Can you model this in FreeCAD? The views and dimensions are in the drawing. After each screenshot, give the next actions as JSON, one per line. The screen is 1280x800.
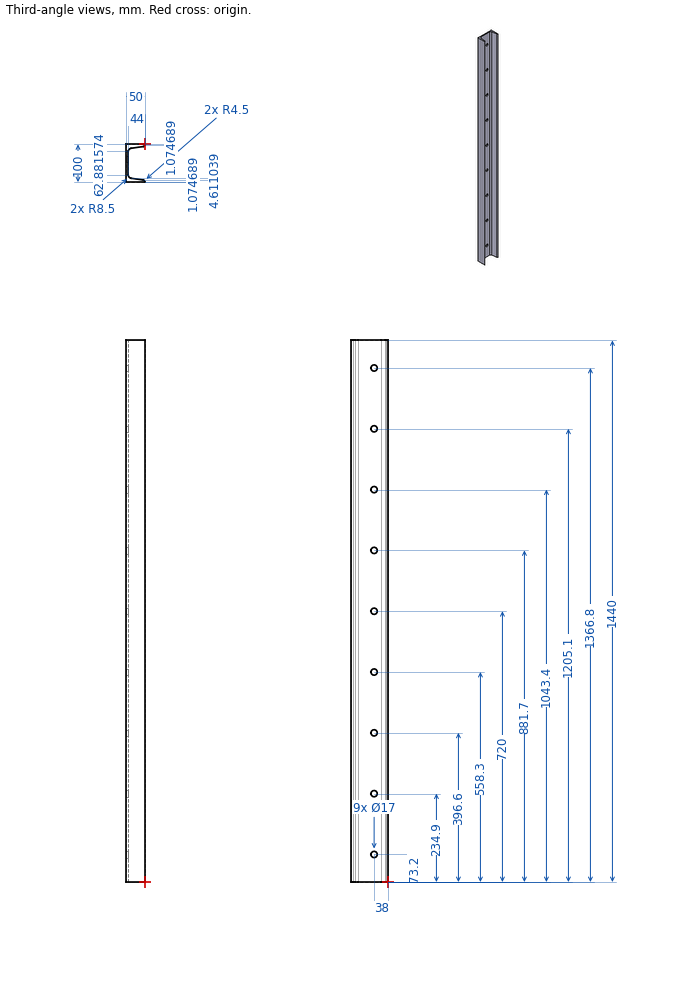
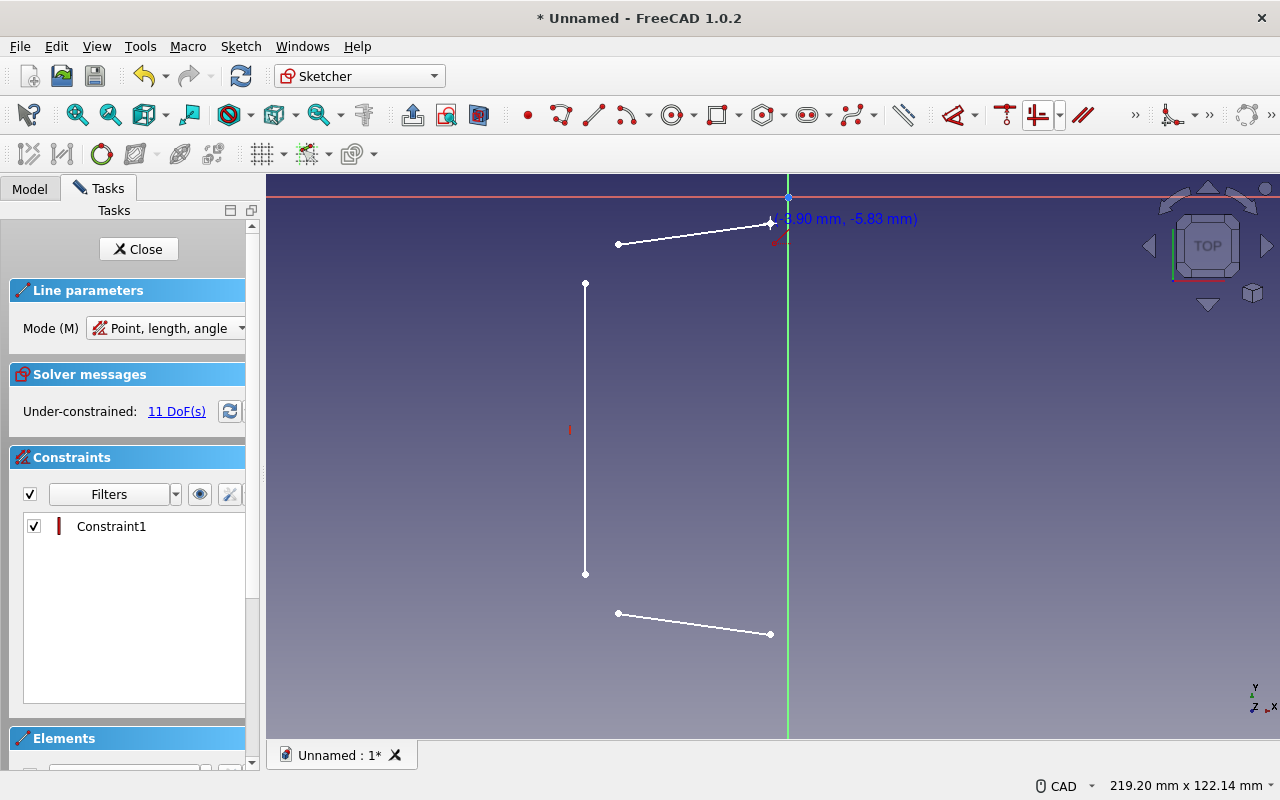
{"action": "left_click", "coordinate": [561, 116]}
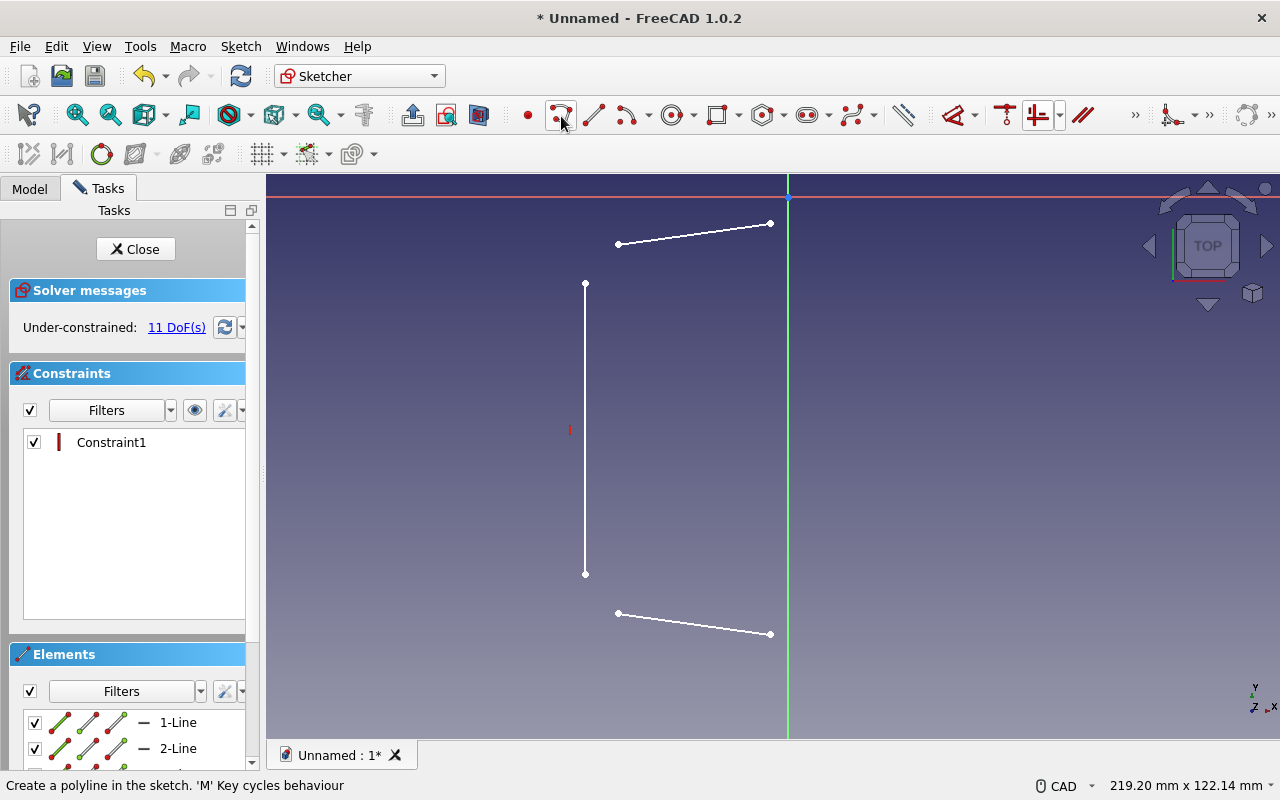
{"action": "scroll", "coordinate": [788, 202], "scroll_direction": "up", "scroll_amount": 6}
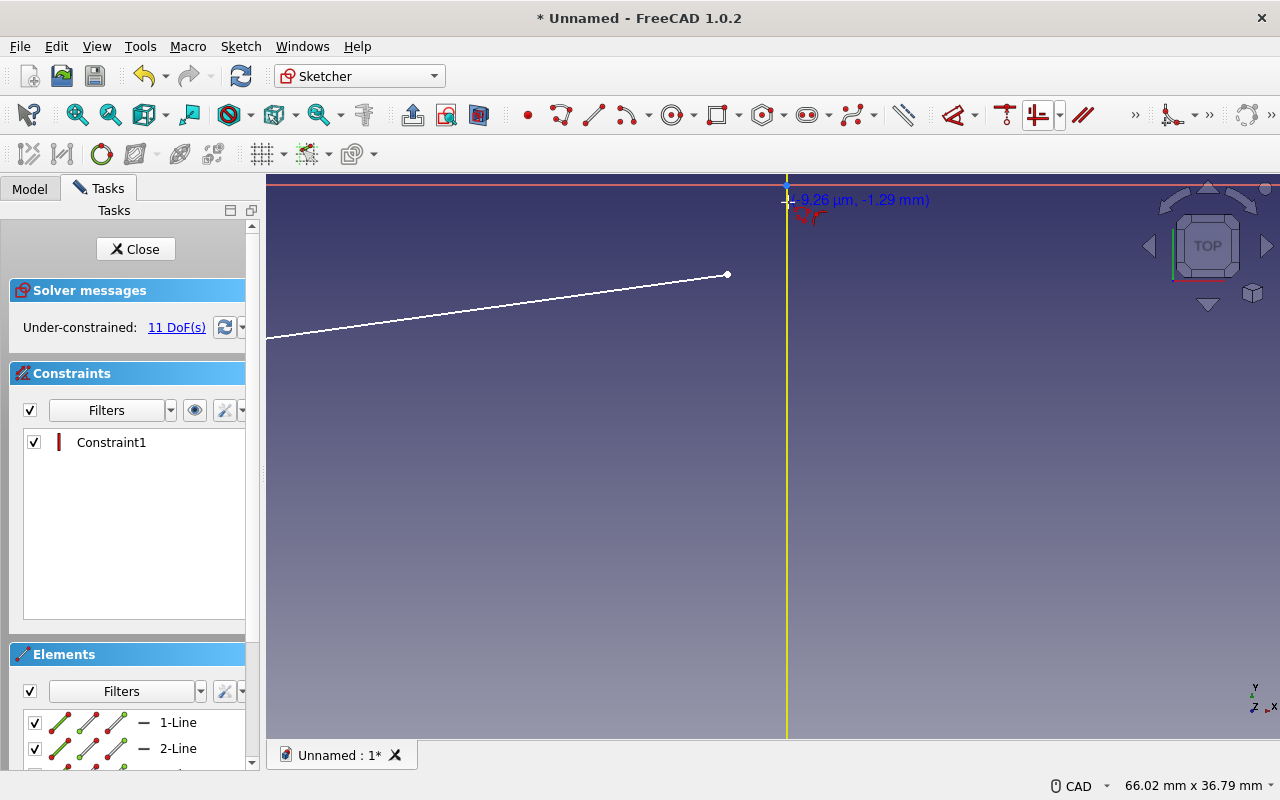
{"action": "left_click", "coordinate": [787, 202]}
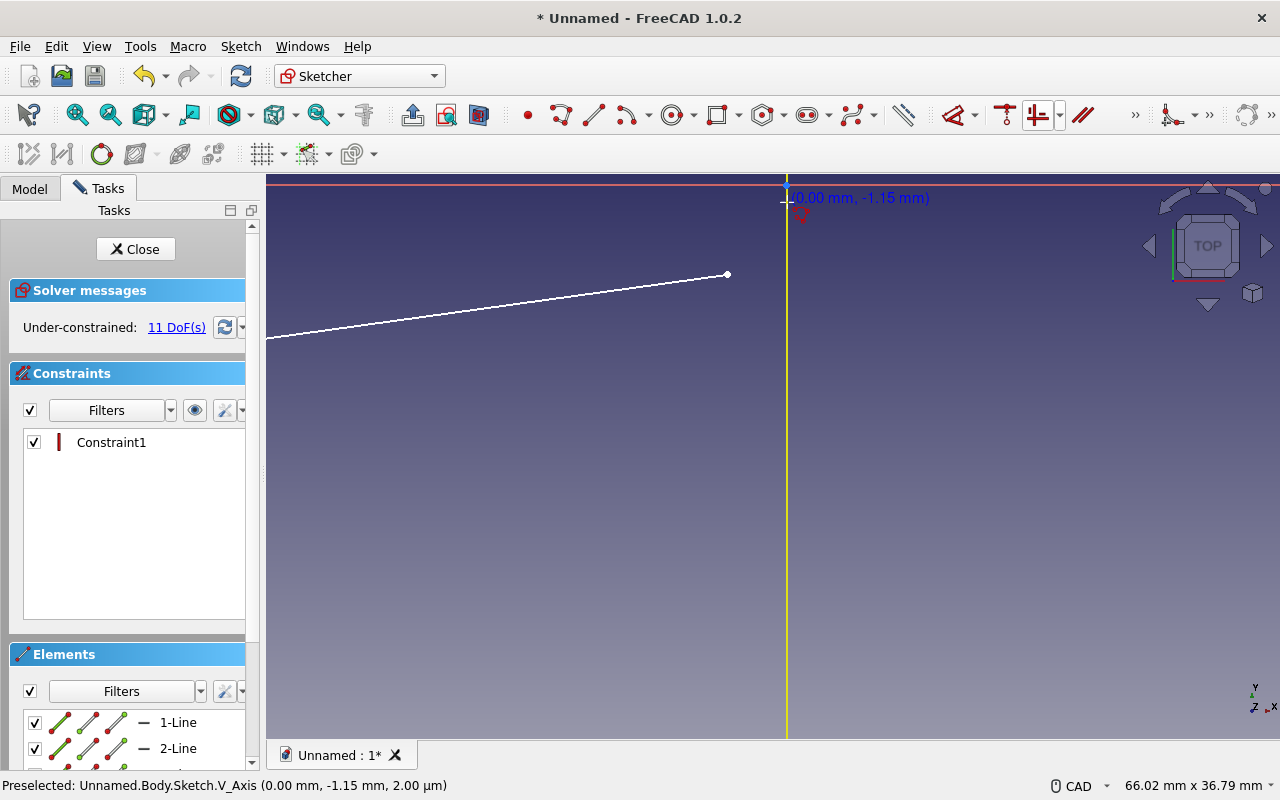
{"action": "scroll", "coordinate": [803, 294], "scroll_direction": "down", "scroll_amount": 7}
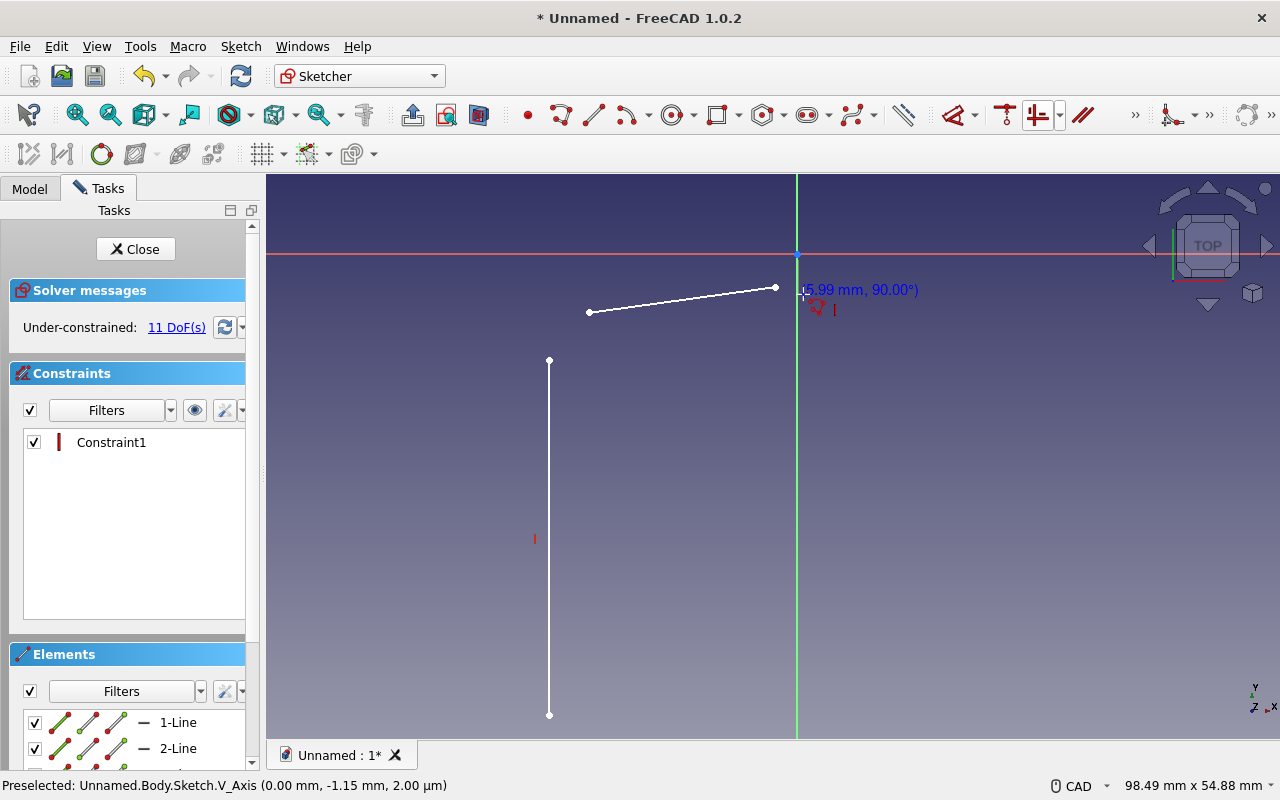
{"action": "scroll", "coordinate": [799, 267], "scroll_direction": "up", "scroll_amount": 7}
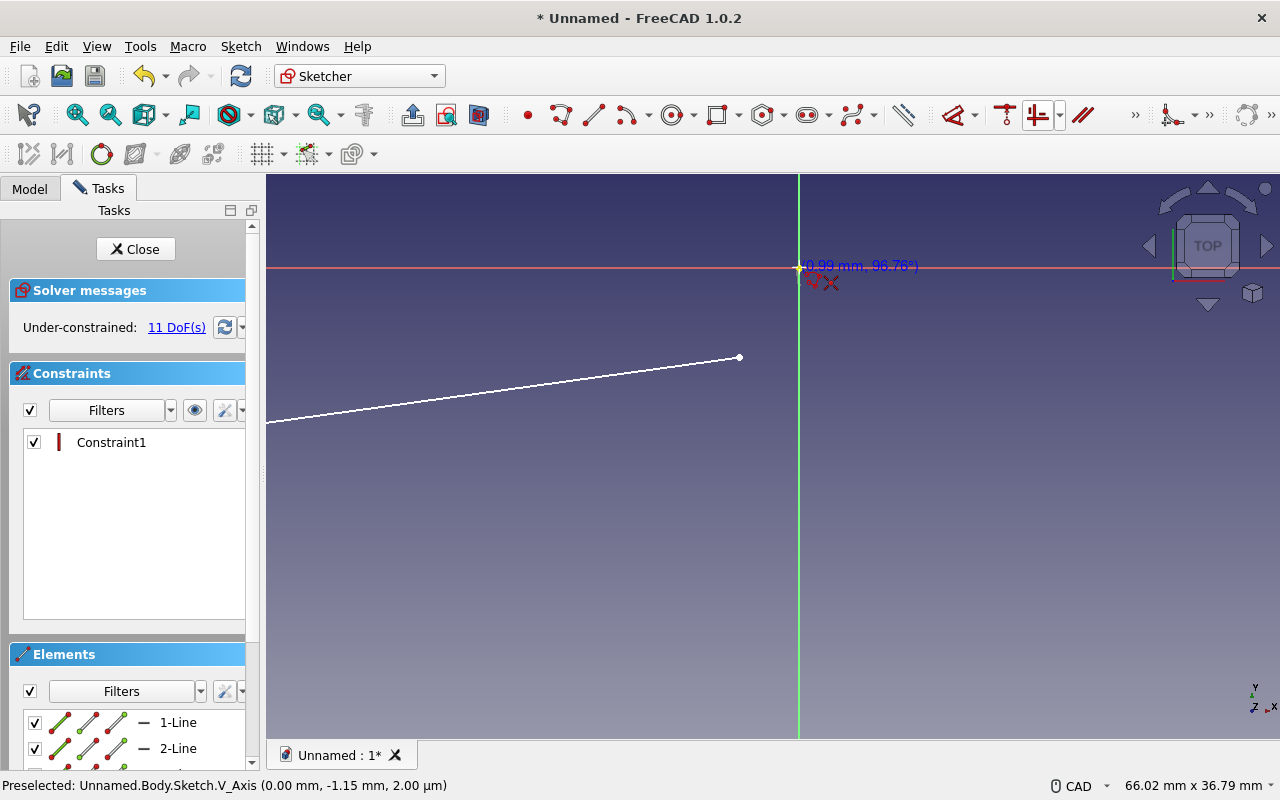
{"action": "left_click", "coordinate": [799, 268]}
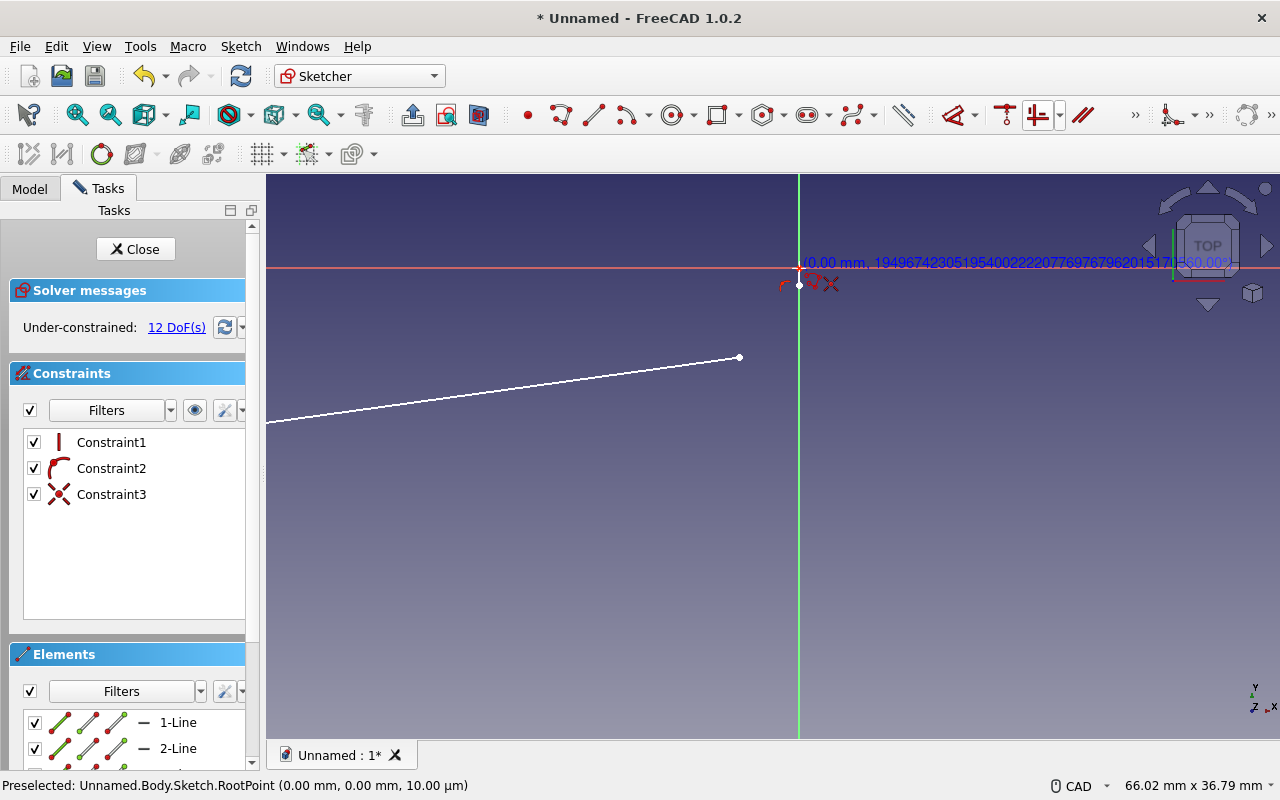
{"action": "scroll", "coordinate": [799, 267], "scroll_direction": "down", "scroll_amount": 7}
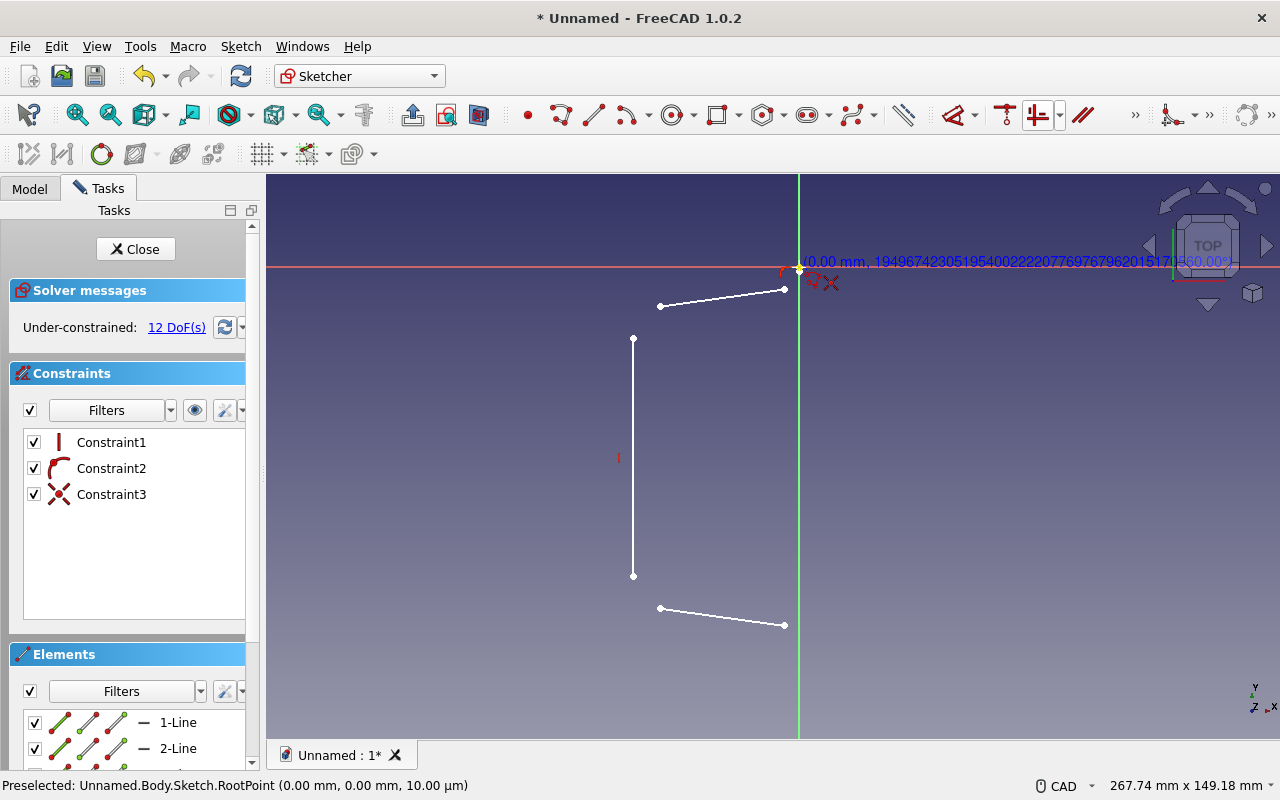
{"action": "left_click", "coordinate": [610, 276]}
{"action": "left_click", "coordinate": [610, 646]}
{"action": "left_click", "coordinate": [799, 646]}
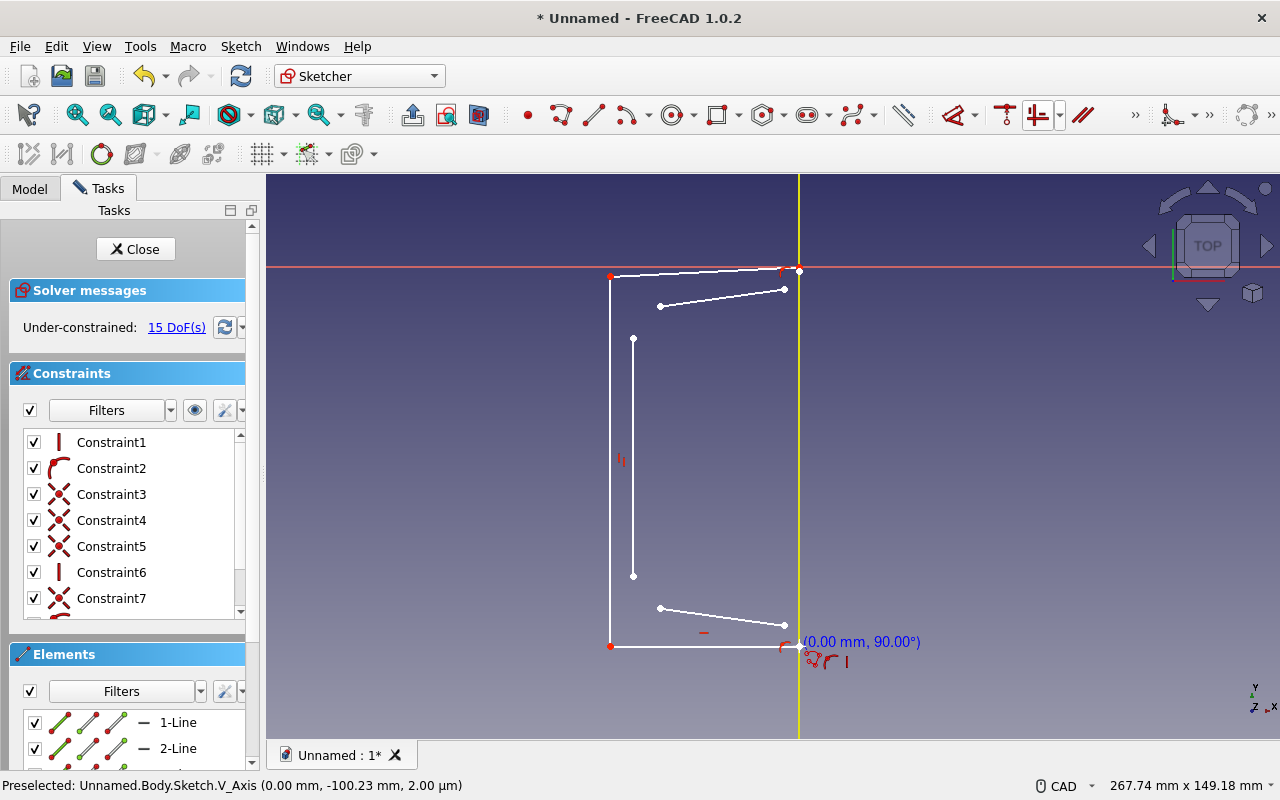
{"action": "scroll", "coordinate": [799, 642], "scroll_direction": "up", "scroll_amount": 7}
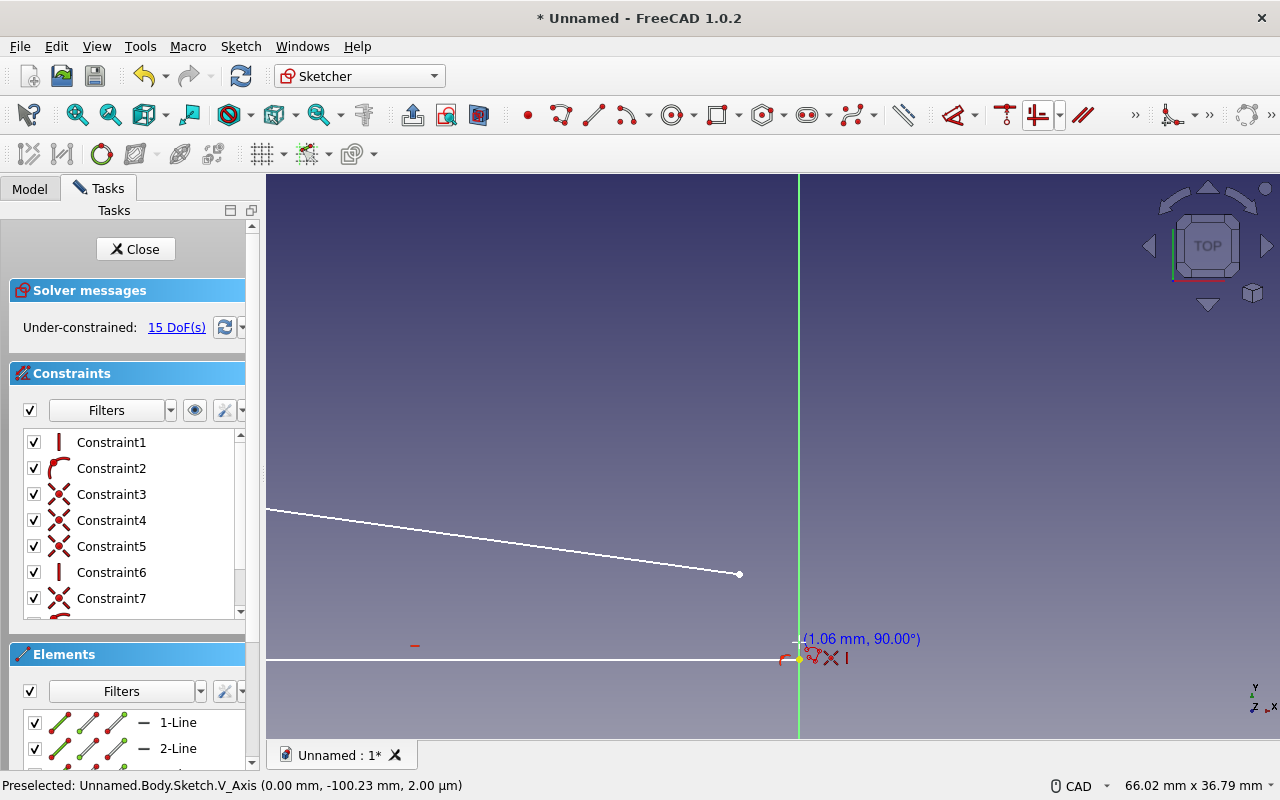
{"action": "left_click", "coordinate": [790, 640]}
{"action": "right_click", "coordinate": [790, 640]}